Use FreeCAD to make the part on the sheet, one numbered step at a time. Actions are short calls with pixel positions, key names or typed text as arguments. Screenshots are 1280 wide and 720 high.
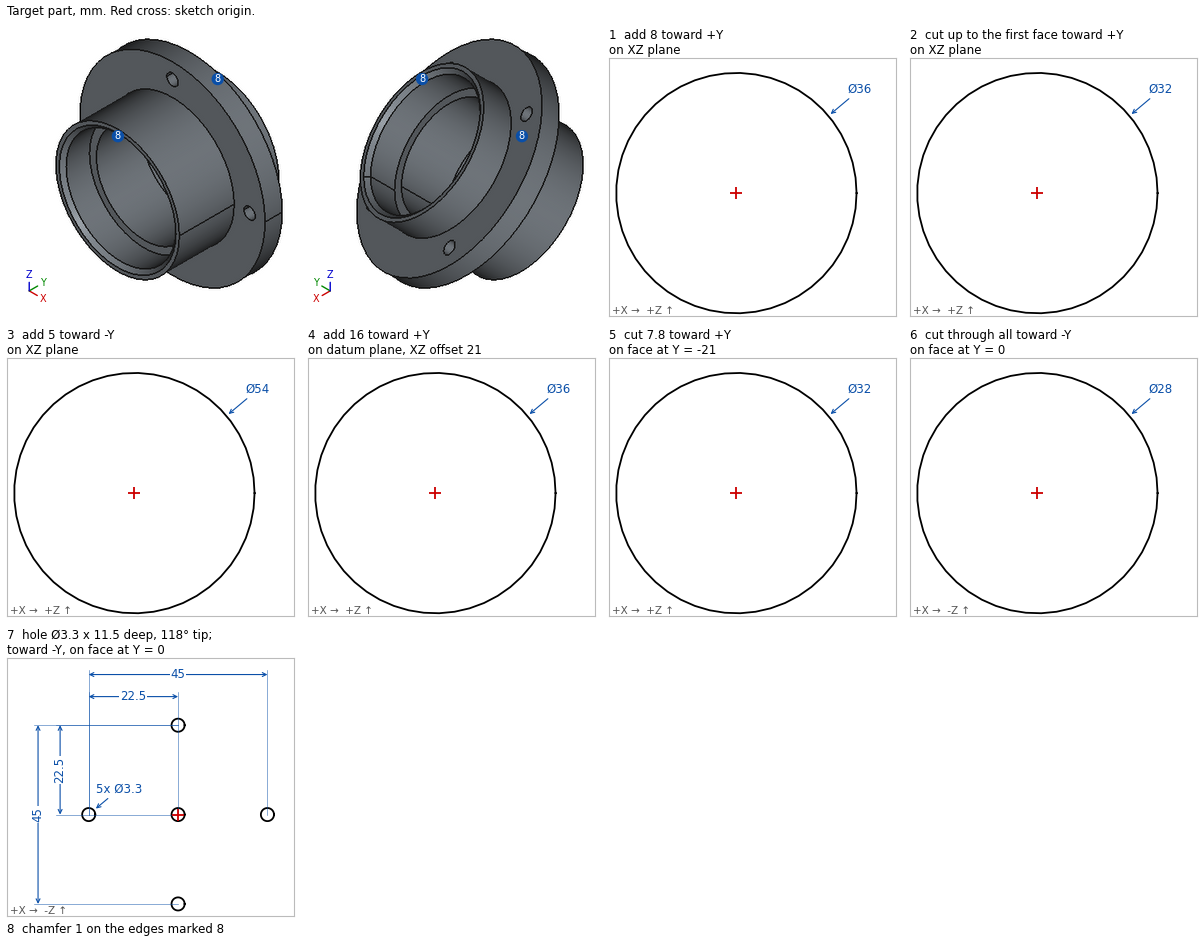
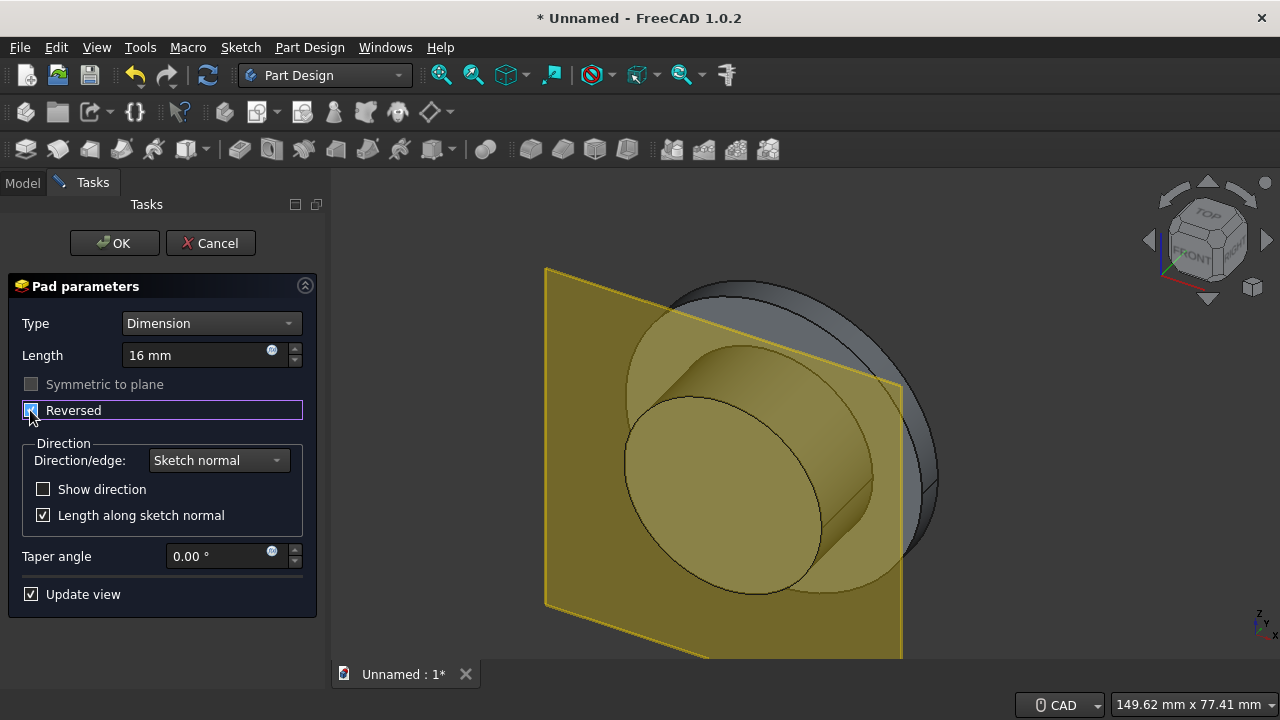
click(115, 243)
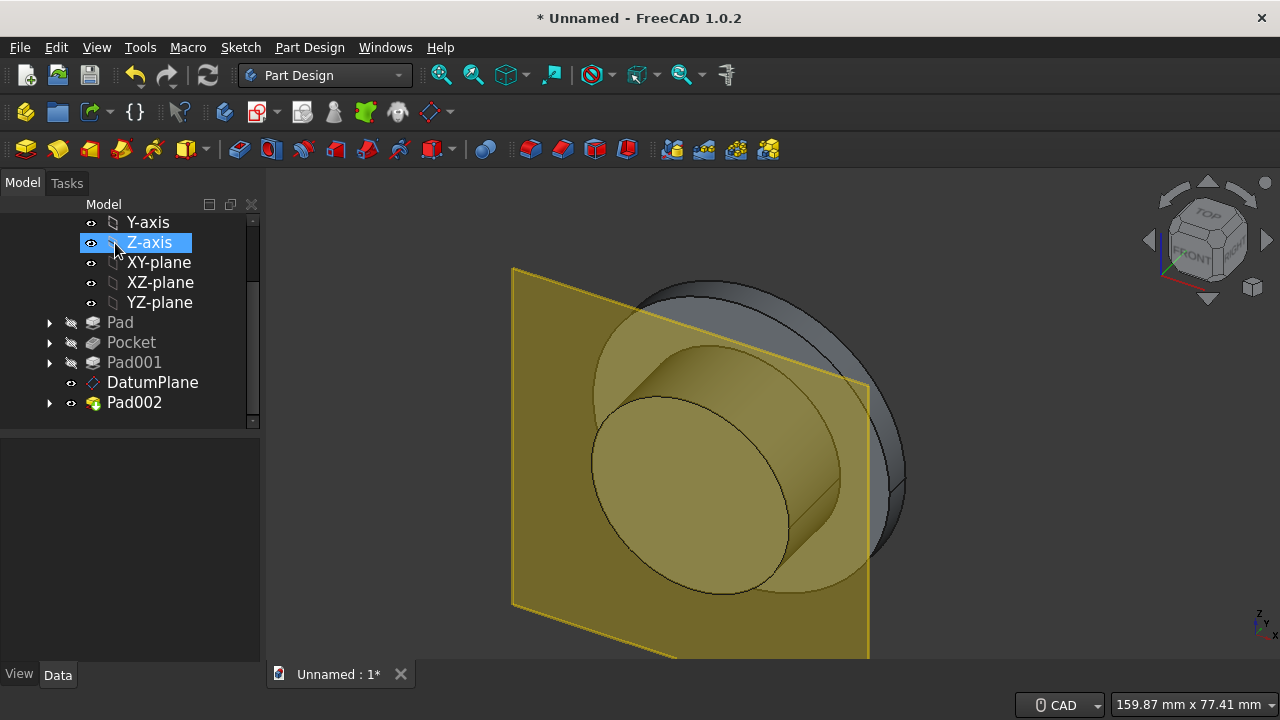
click(116, 383)
key(space)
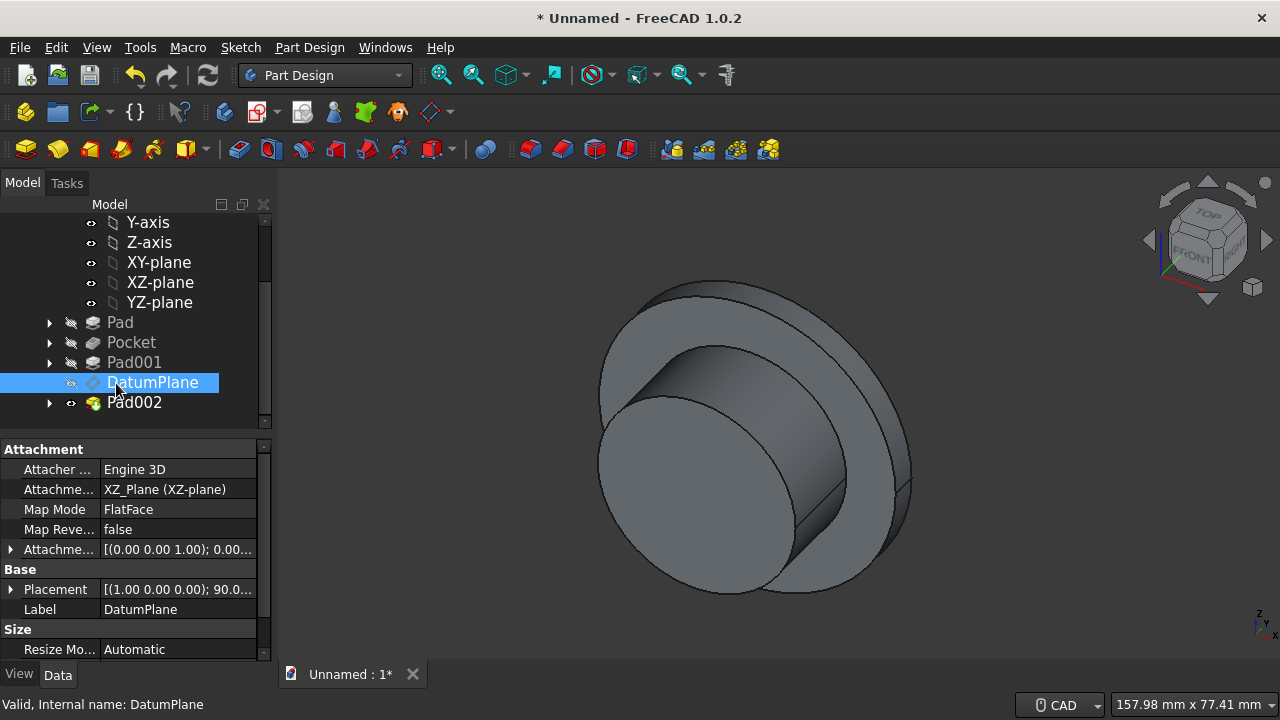
click(442, 76)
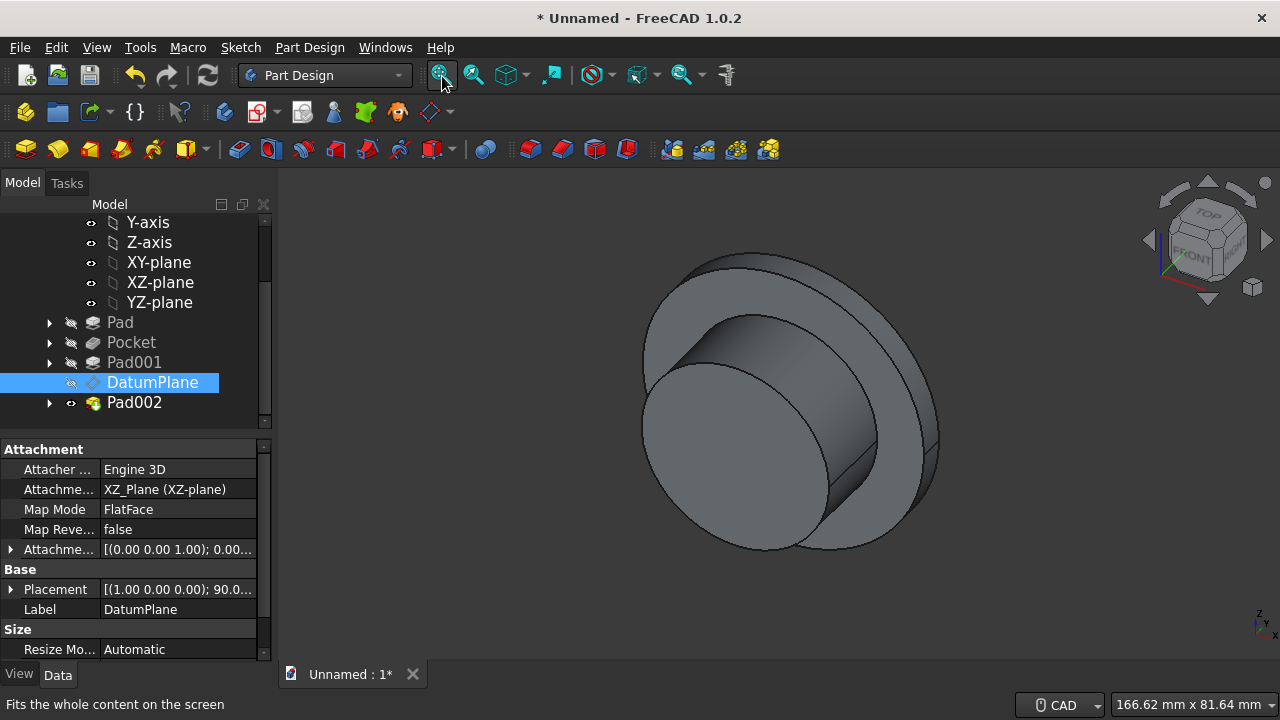
click(735, 456)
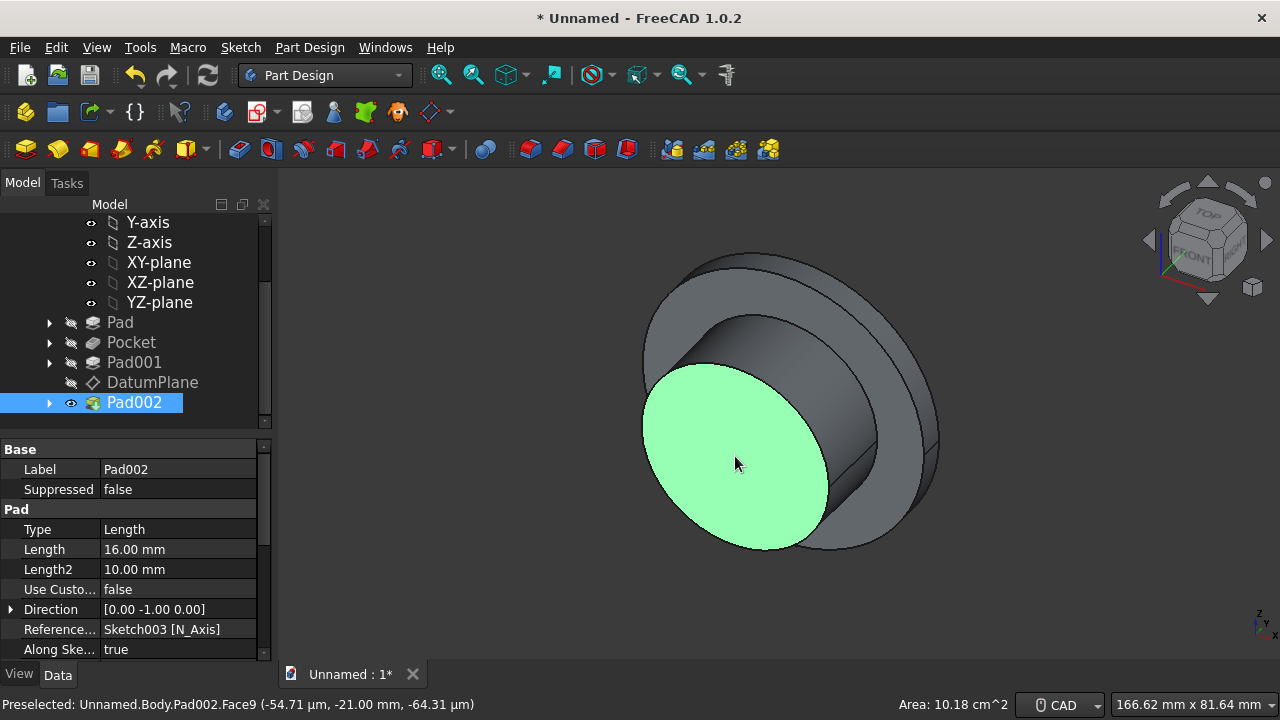
click(258, 112)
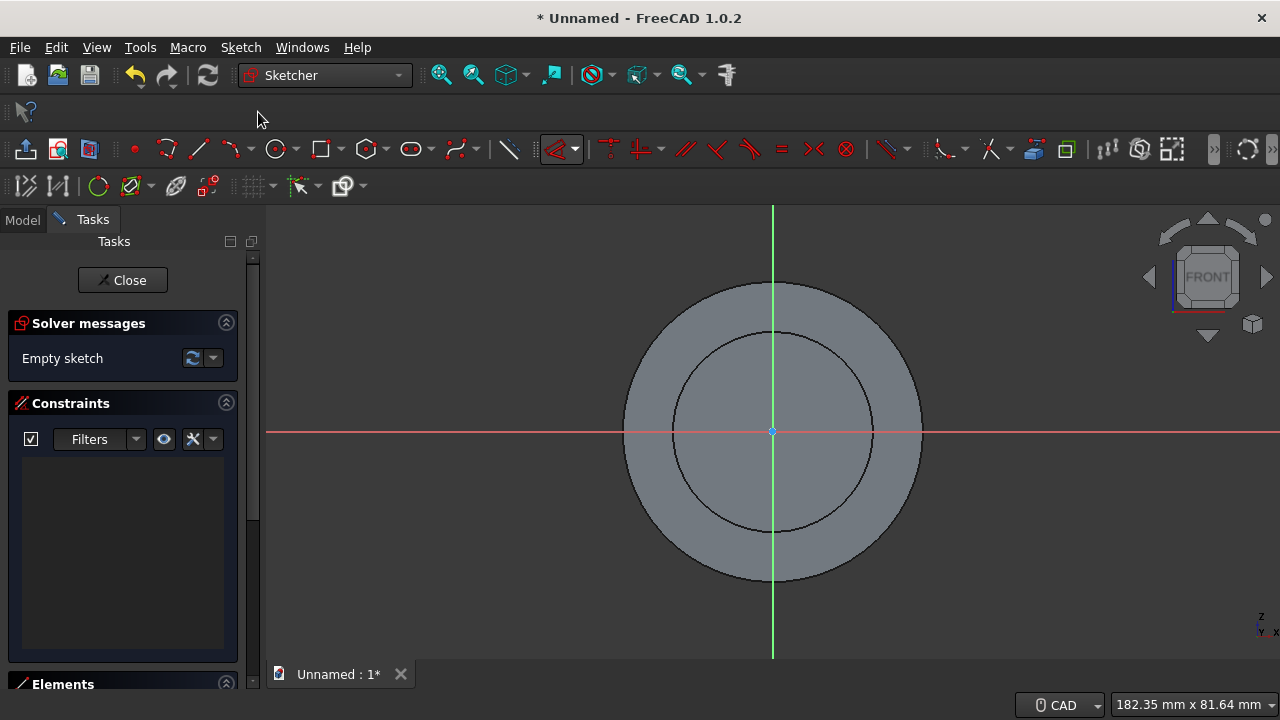
scroll(912, 432, up, 2)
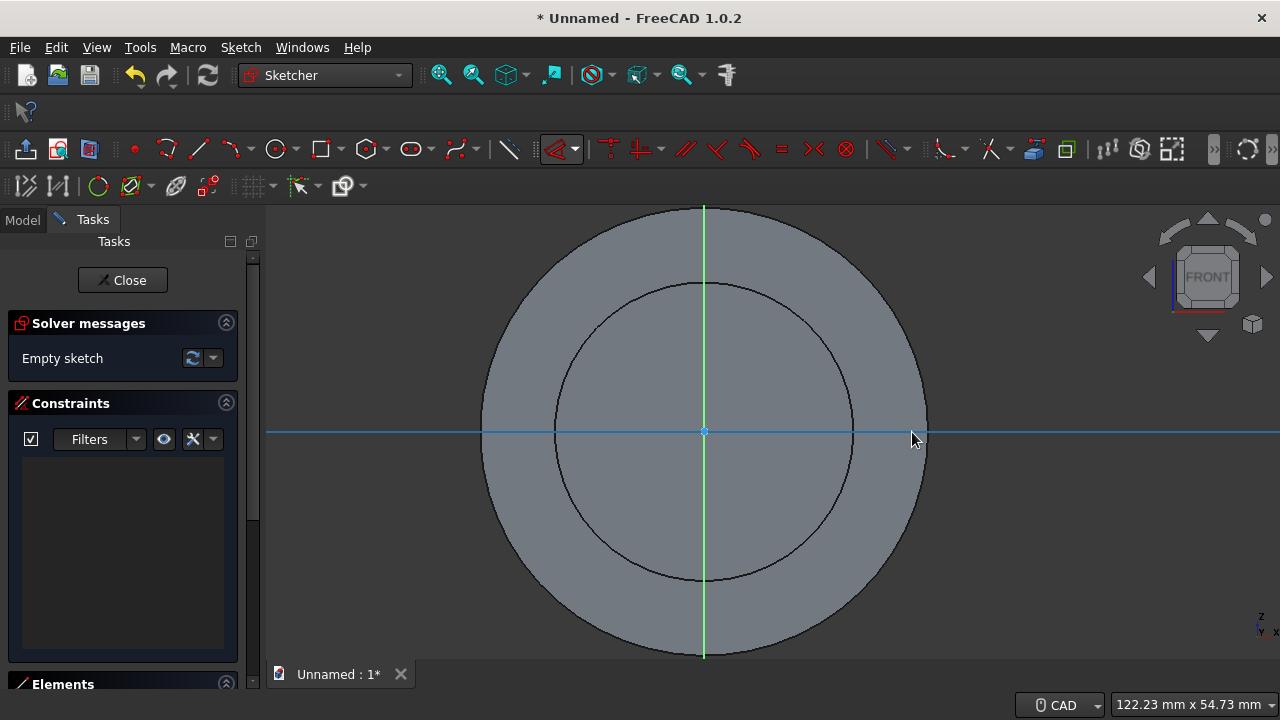
click(276, 150)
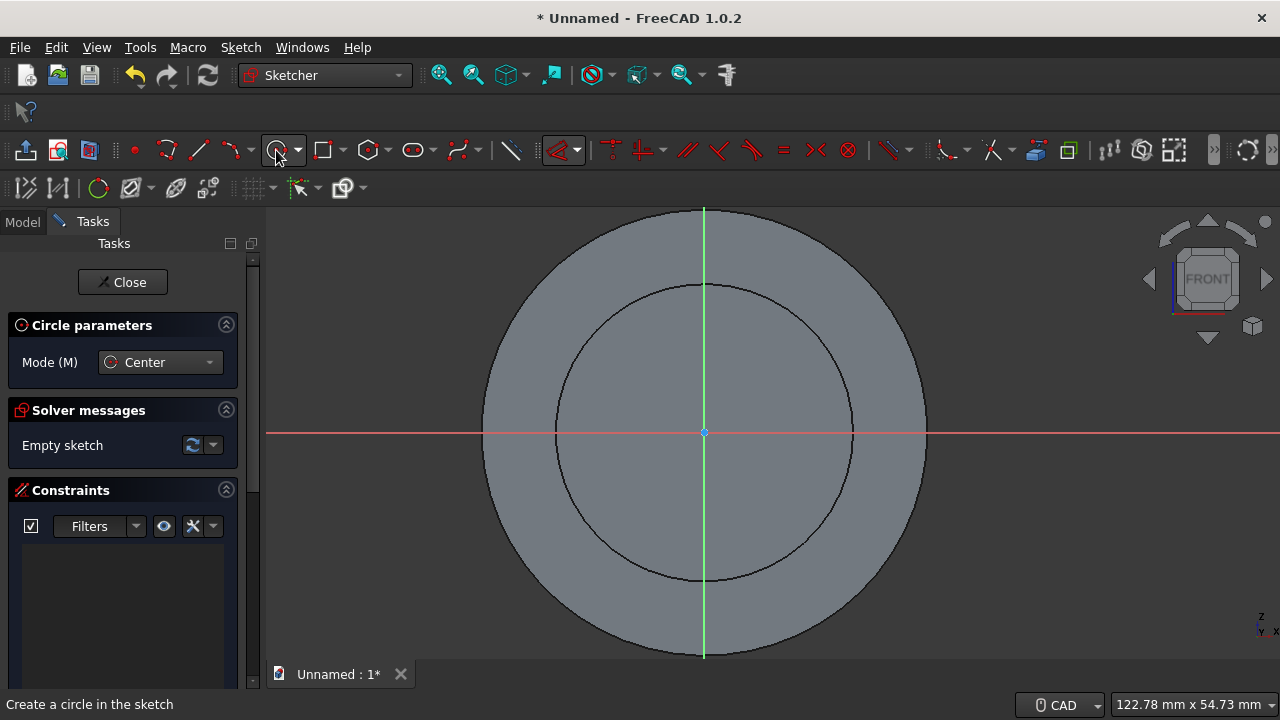
click(704, 433)
click(798, 339)
key(Escape)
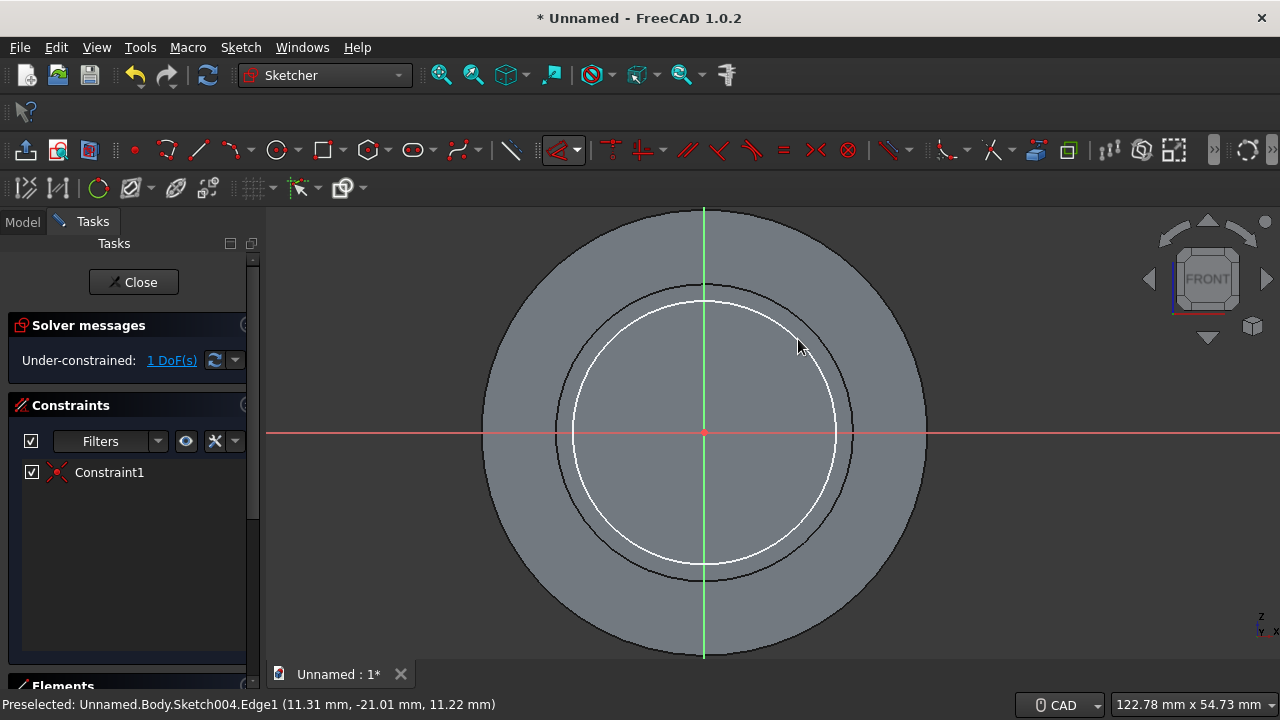
click(797, 339)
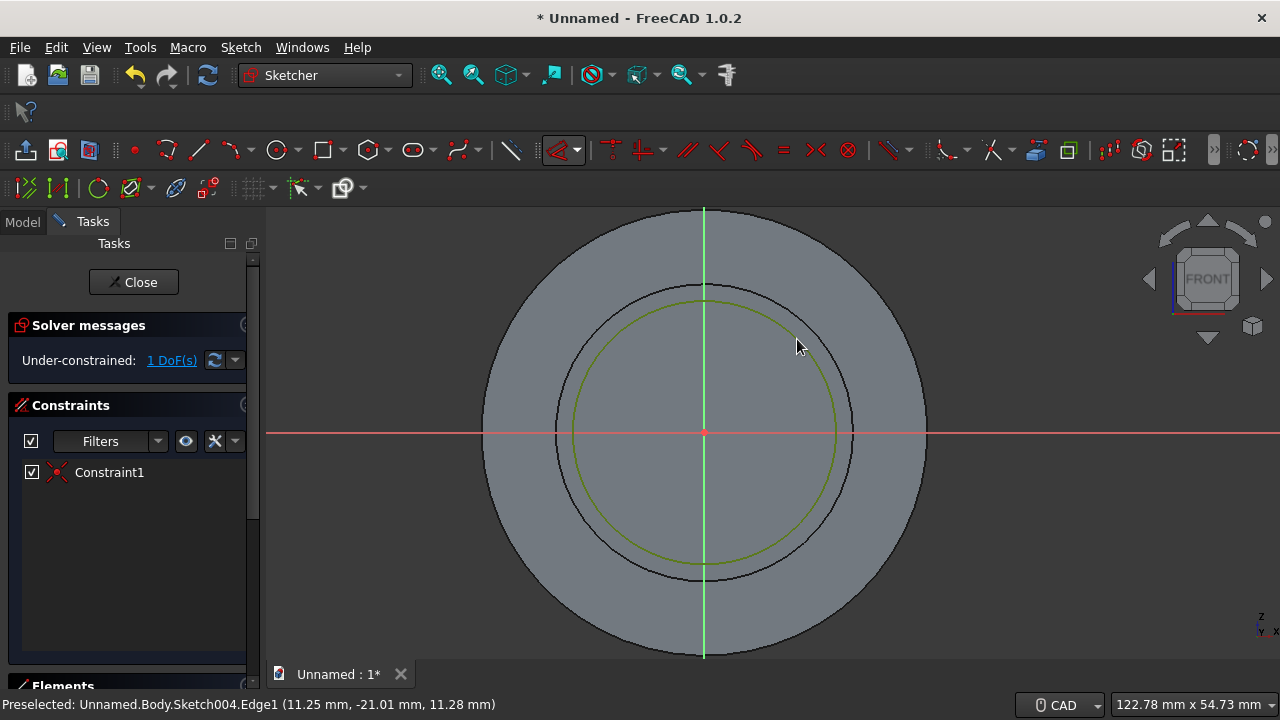
click(580, 150)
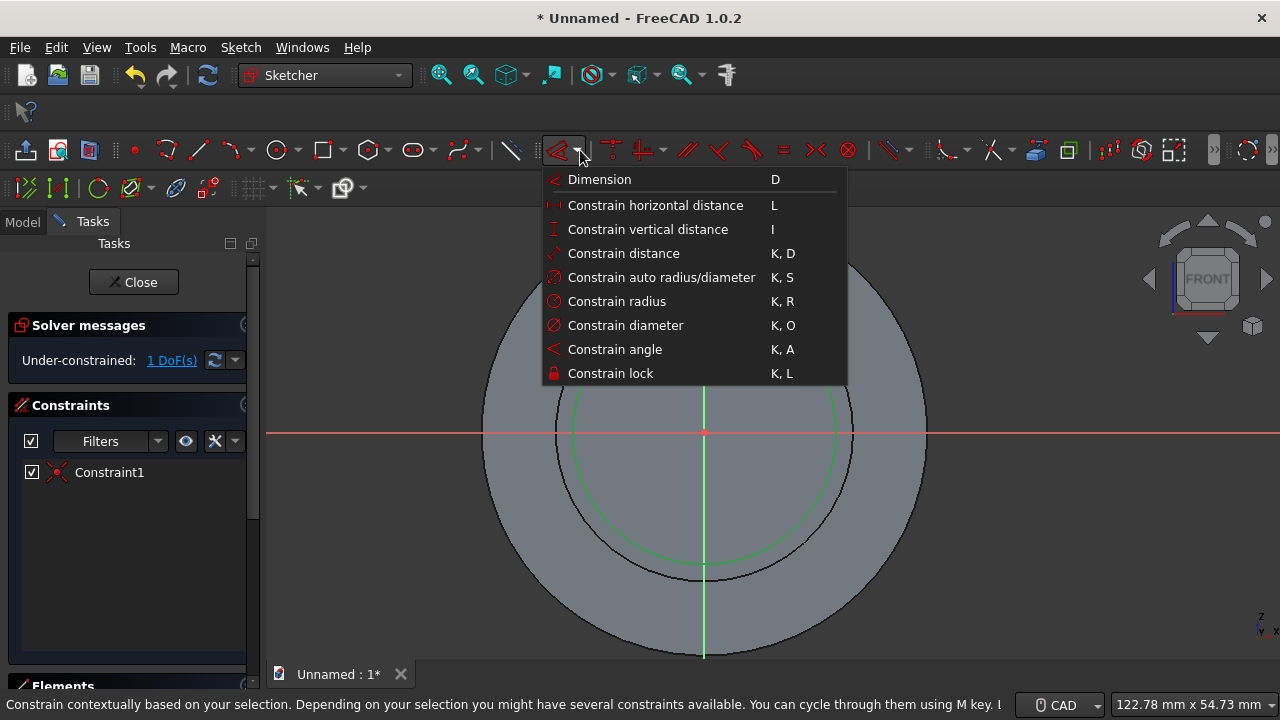
click(695, 325)